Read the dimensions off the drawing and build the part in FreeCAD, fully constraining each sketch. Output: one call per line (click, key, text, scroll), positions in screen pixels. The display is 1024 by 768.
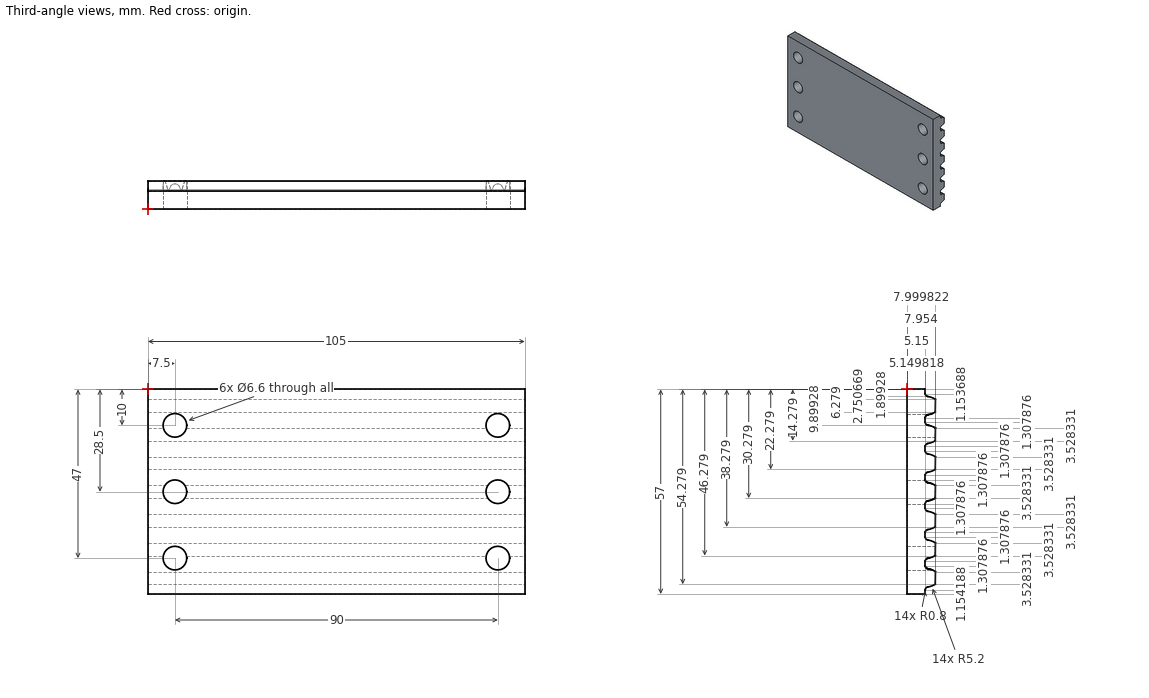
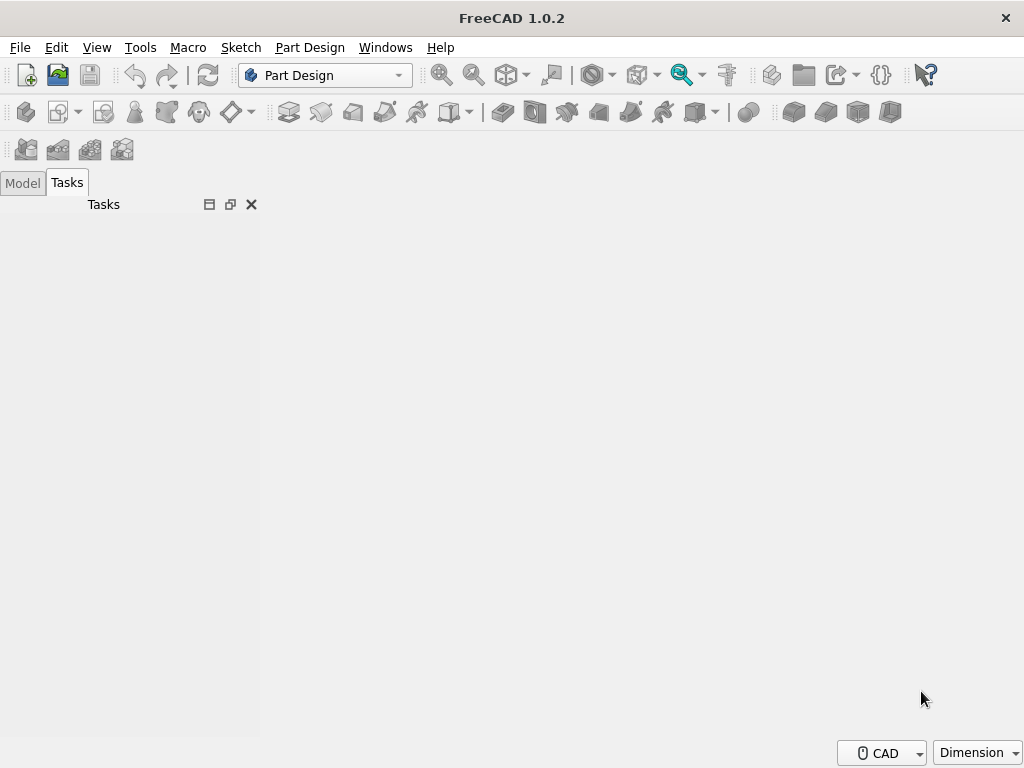
click(26, 76)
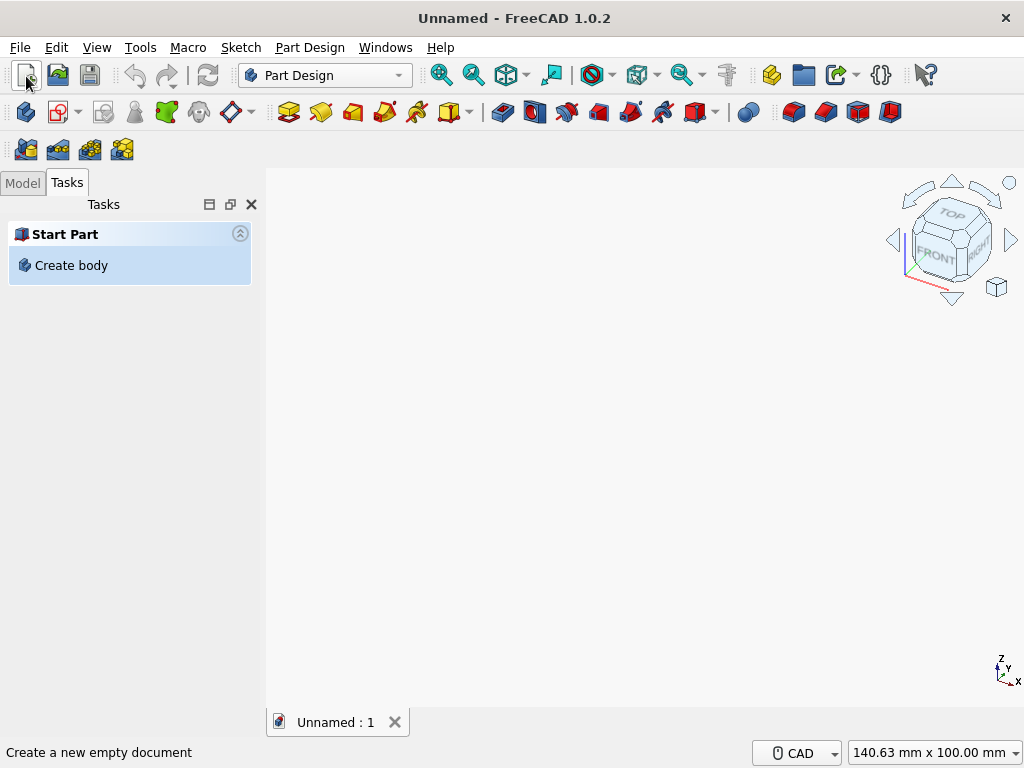
click(58, 112)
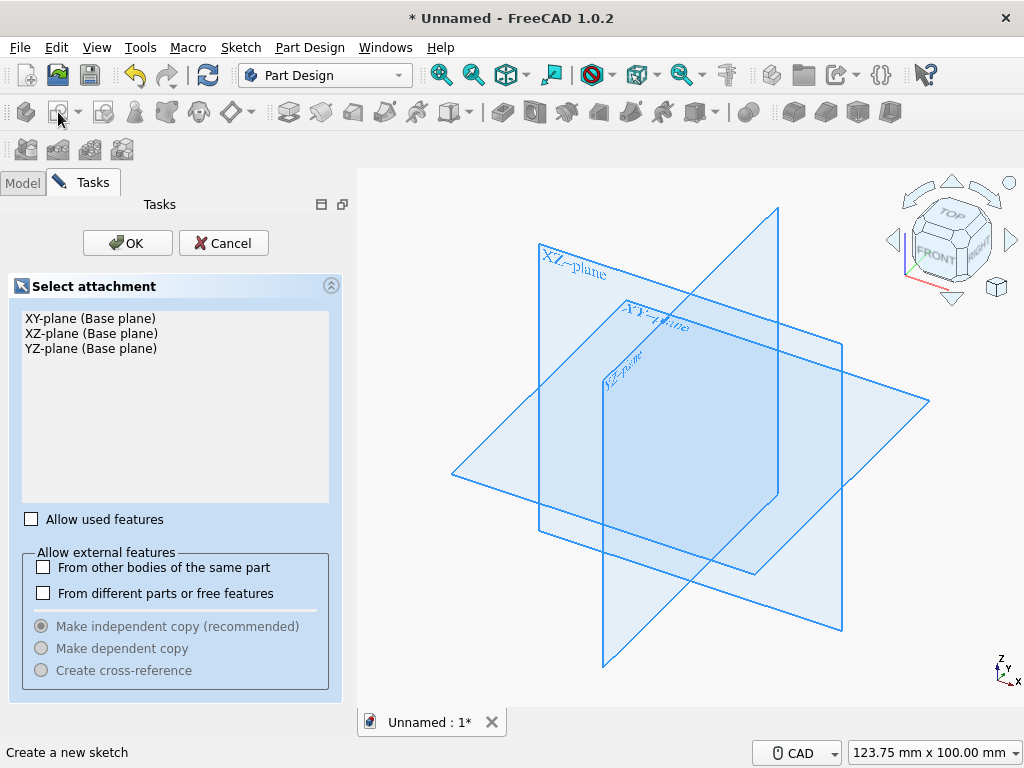
click(82, 348)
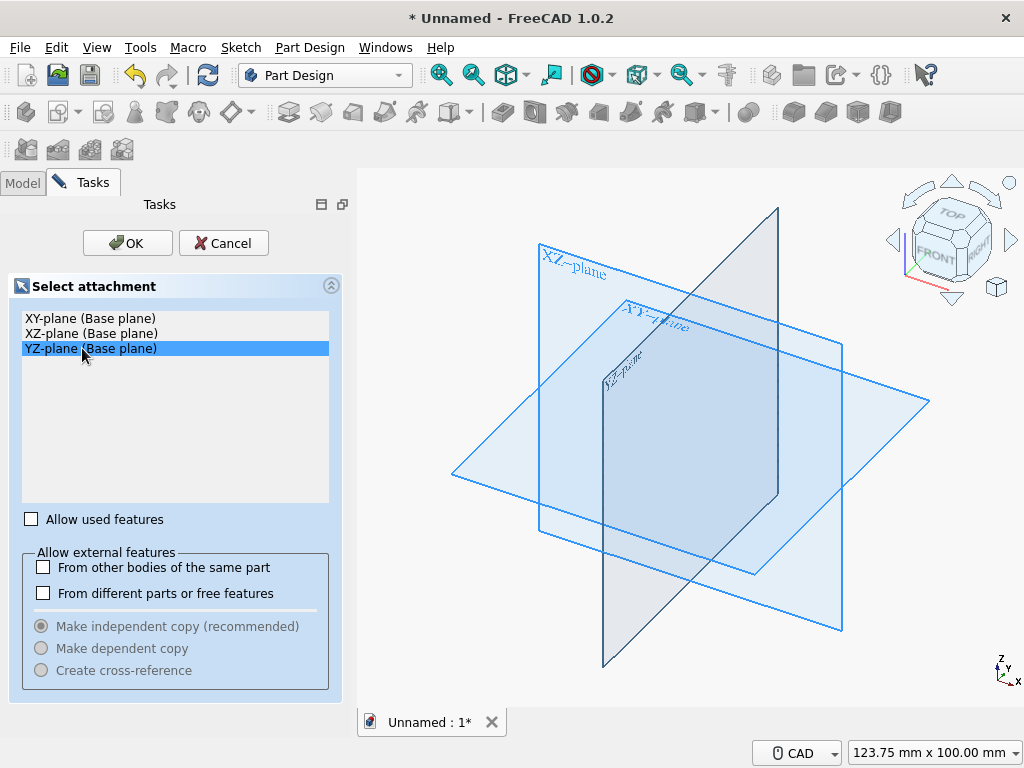
click(128, 243)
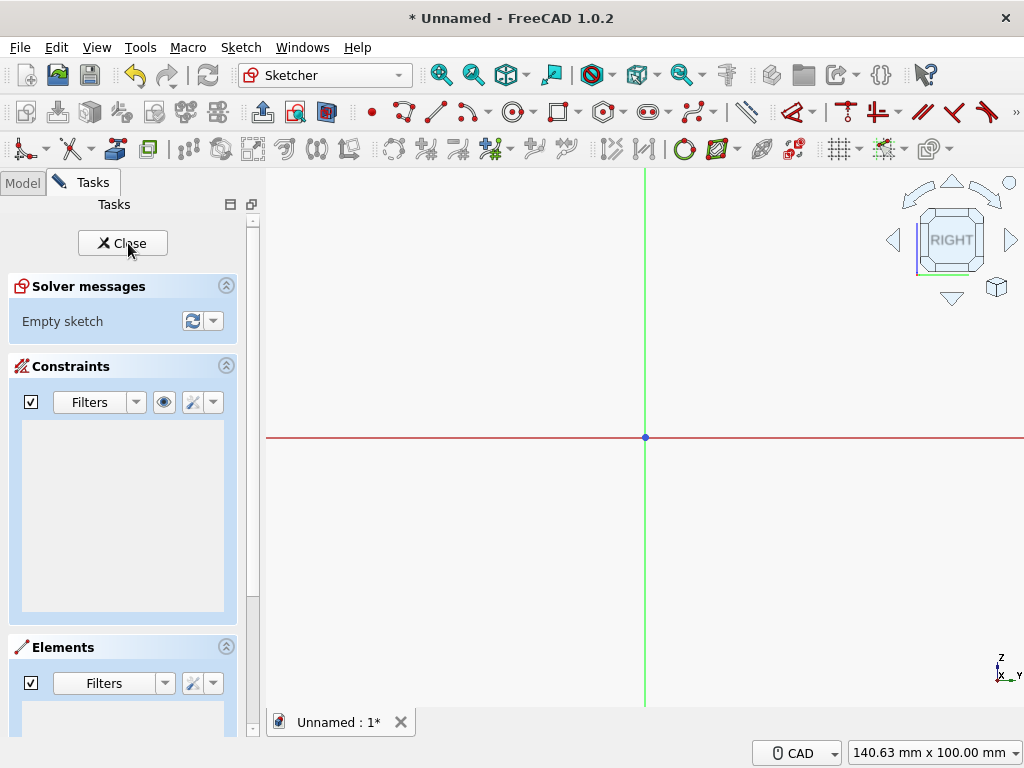
scroll(294, 196, down, 1)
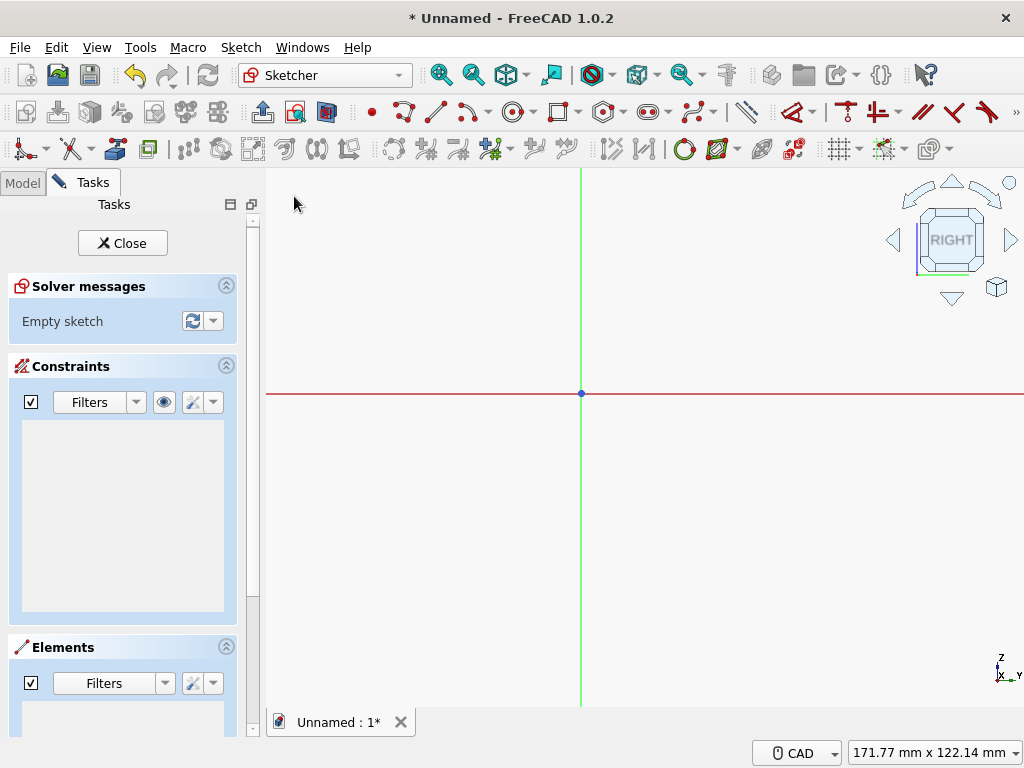
scroll(645, 679, up, 2)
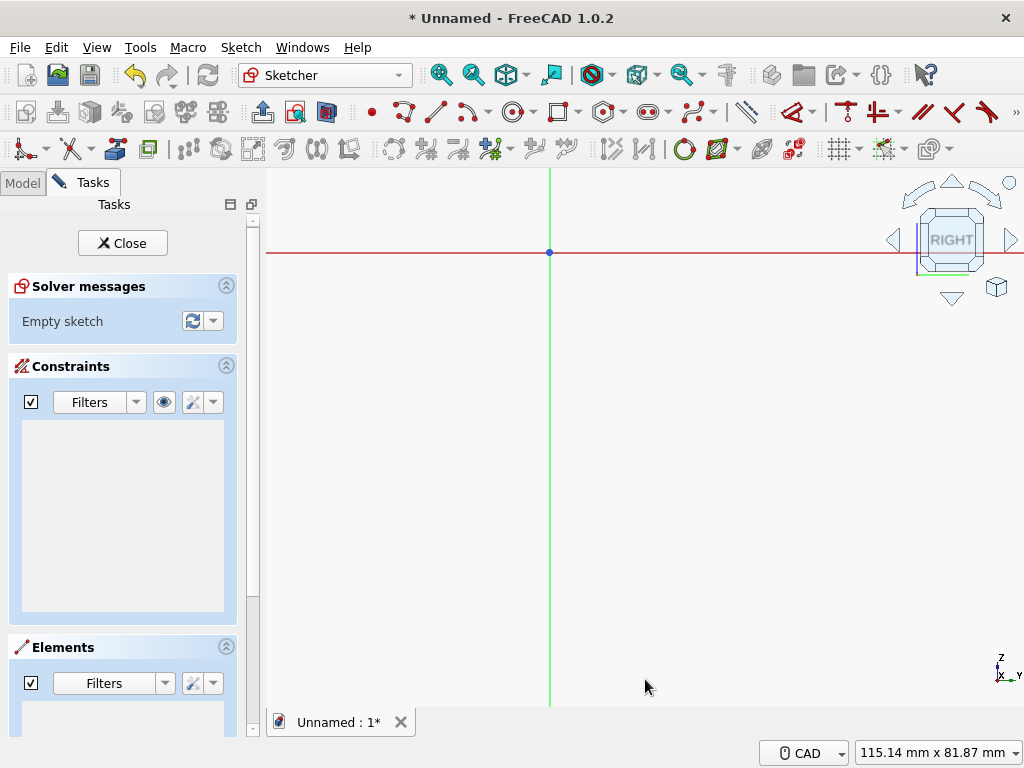
click(404, 112)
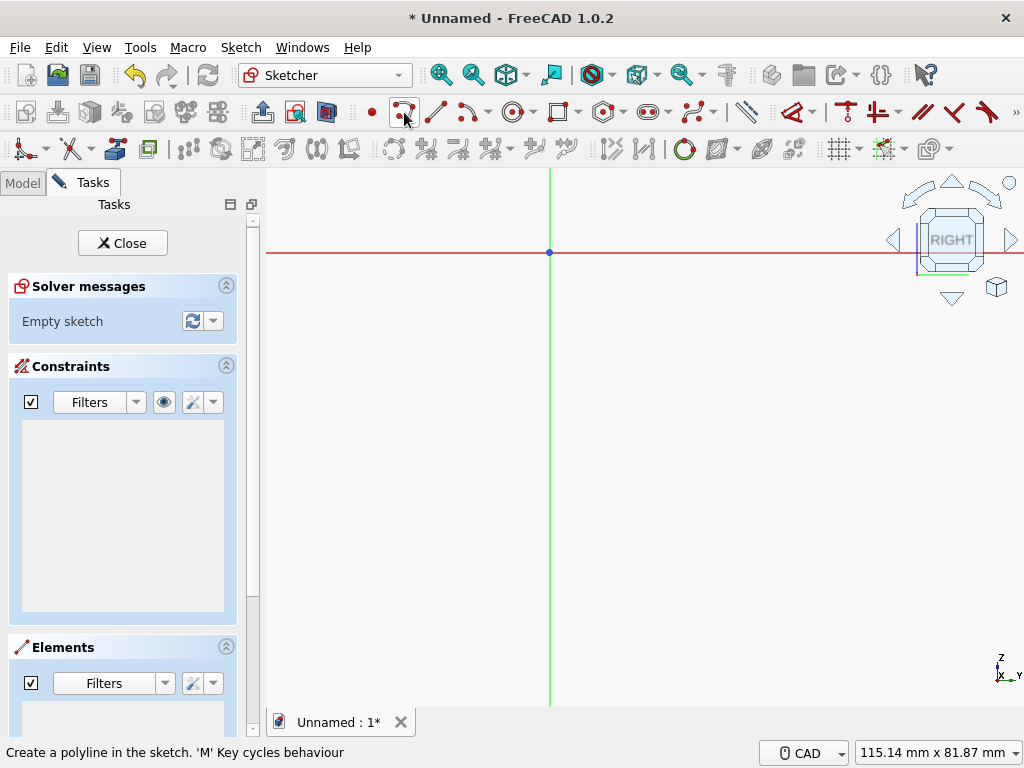
scroll(584, 261, up, 4)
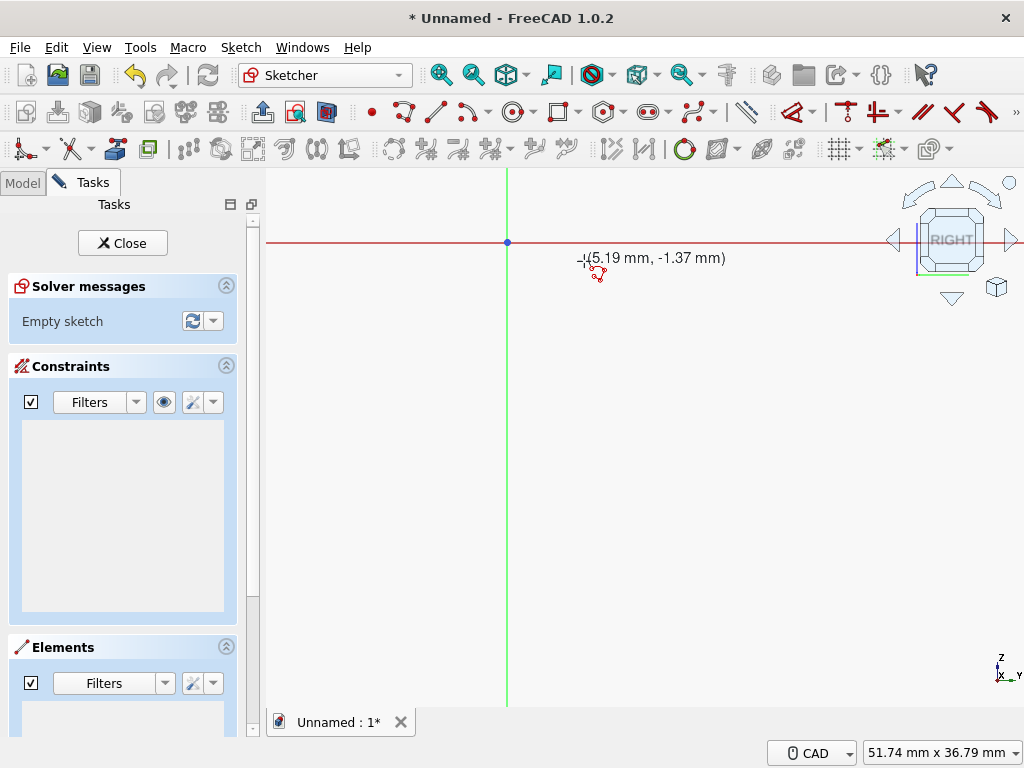
click(583, 260)
click(583, 243)
click(507, 243)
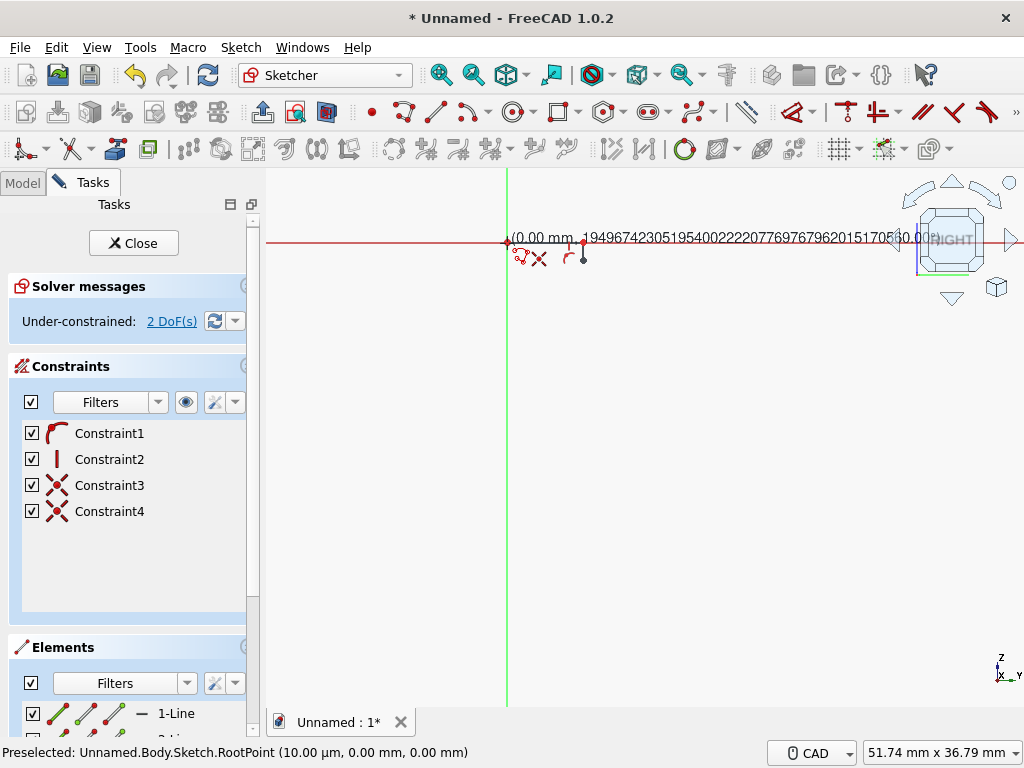
scroll(585, 256, down, 4)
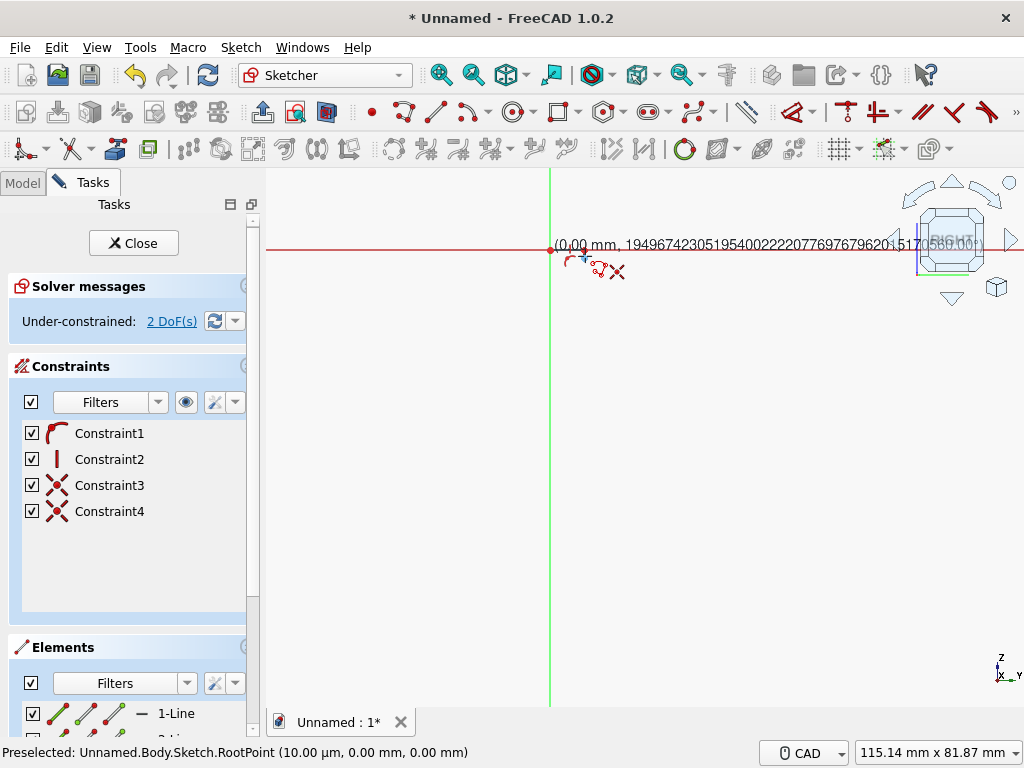
click(559, 625)
click(584, 625)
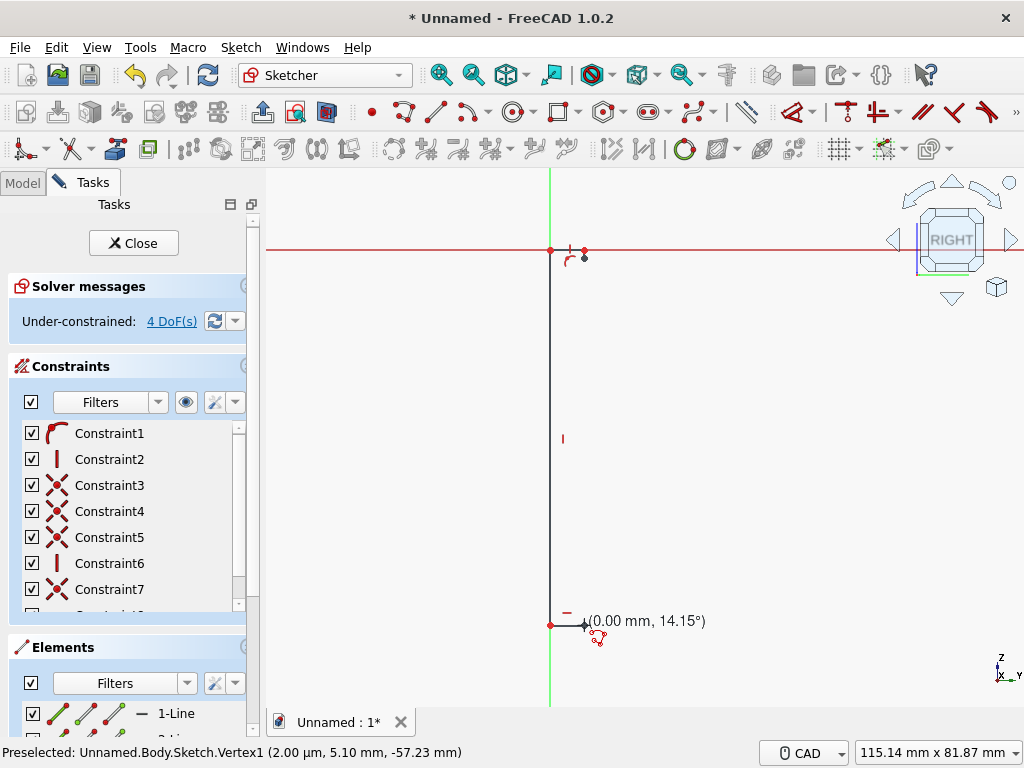
scroll(584, 618, up, 4)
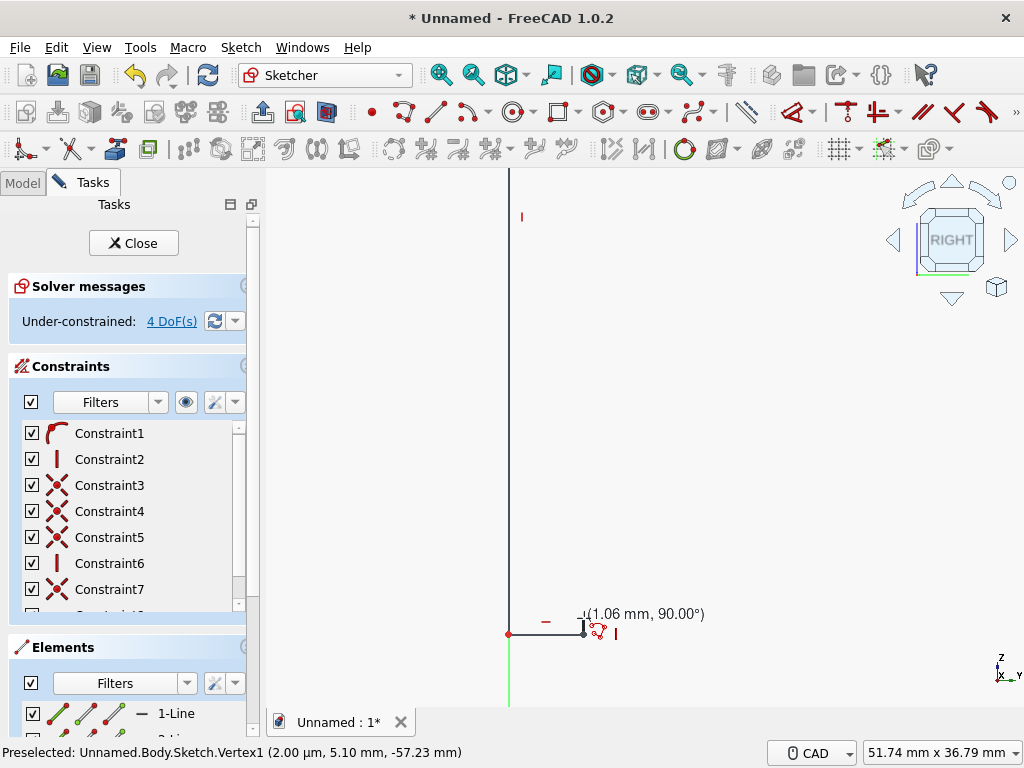
click(583, 617)
right_click(583, 617)